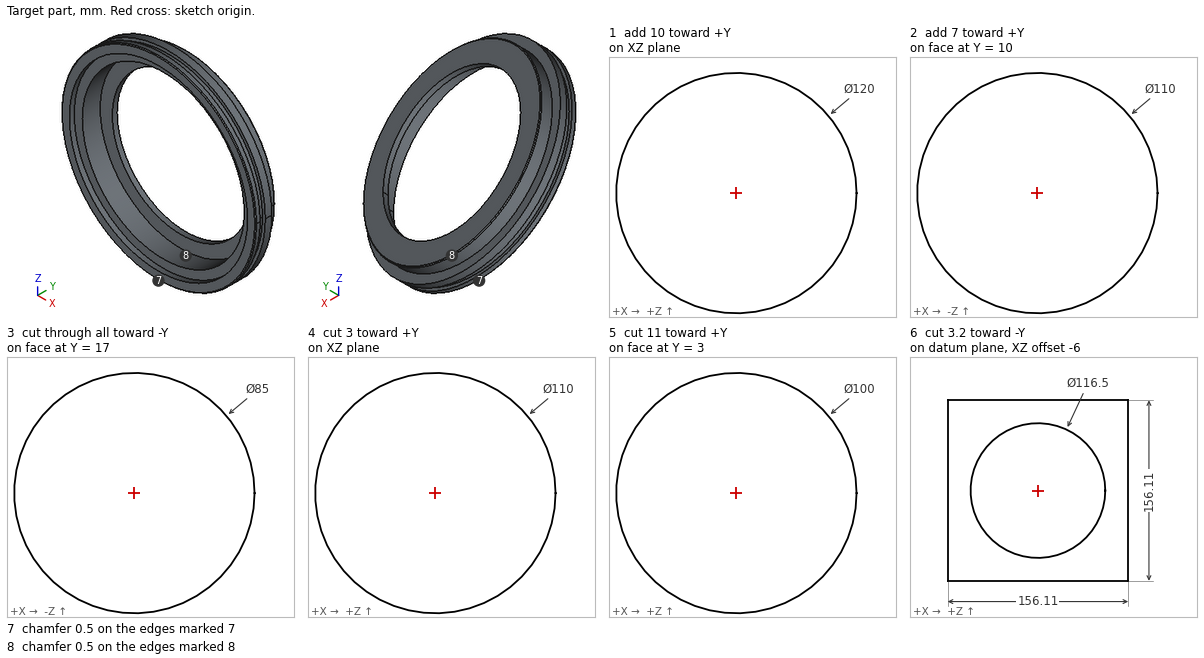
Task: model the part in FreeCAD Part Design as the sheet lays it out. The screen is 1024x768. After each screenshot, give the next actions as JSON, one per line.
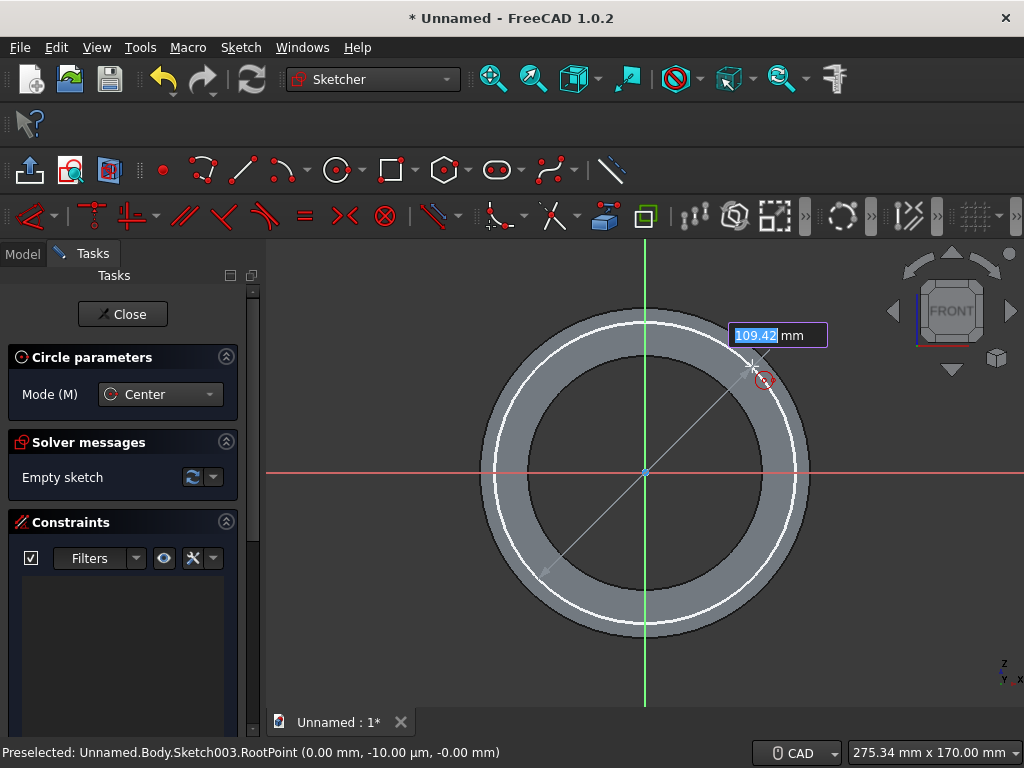
{"action": "type", "text": "110"}
{"action": "key", "text": "Return"}
{"action": "key", "text": "Escape"}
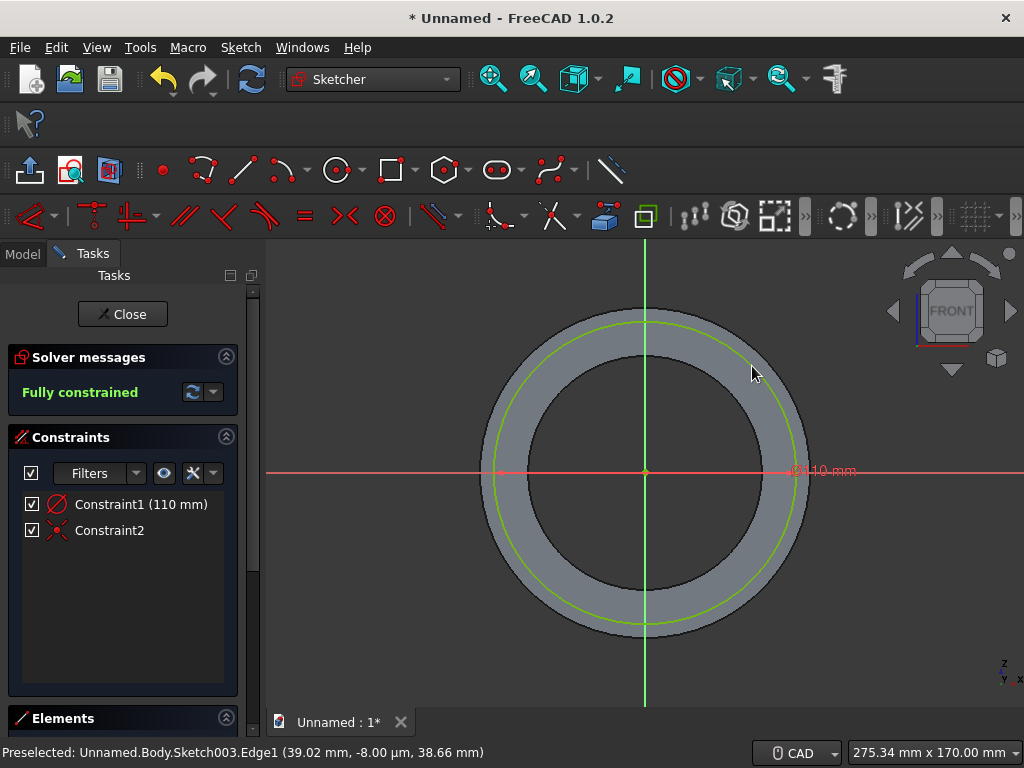
{"action": "left_click", "coordinate": [123, 314]}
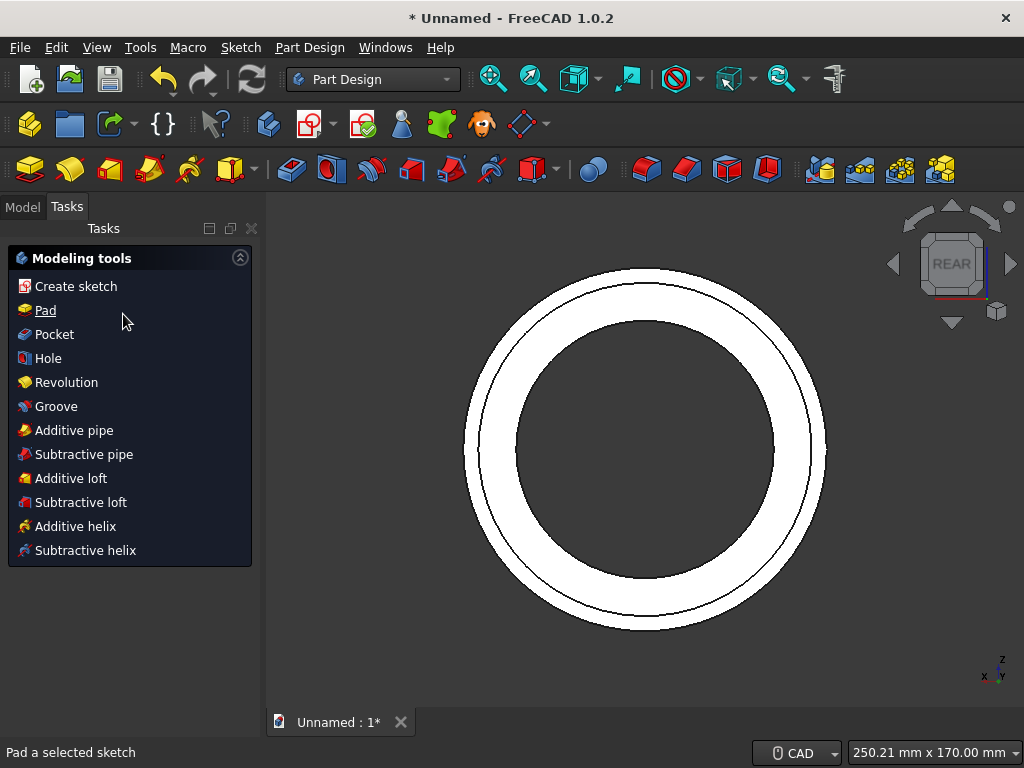
{"action": "left_click", "coordinate": [292, 170]}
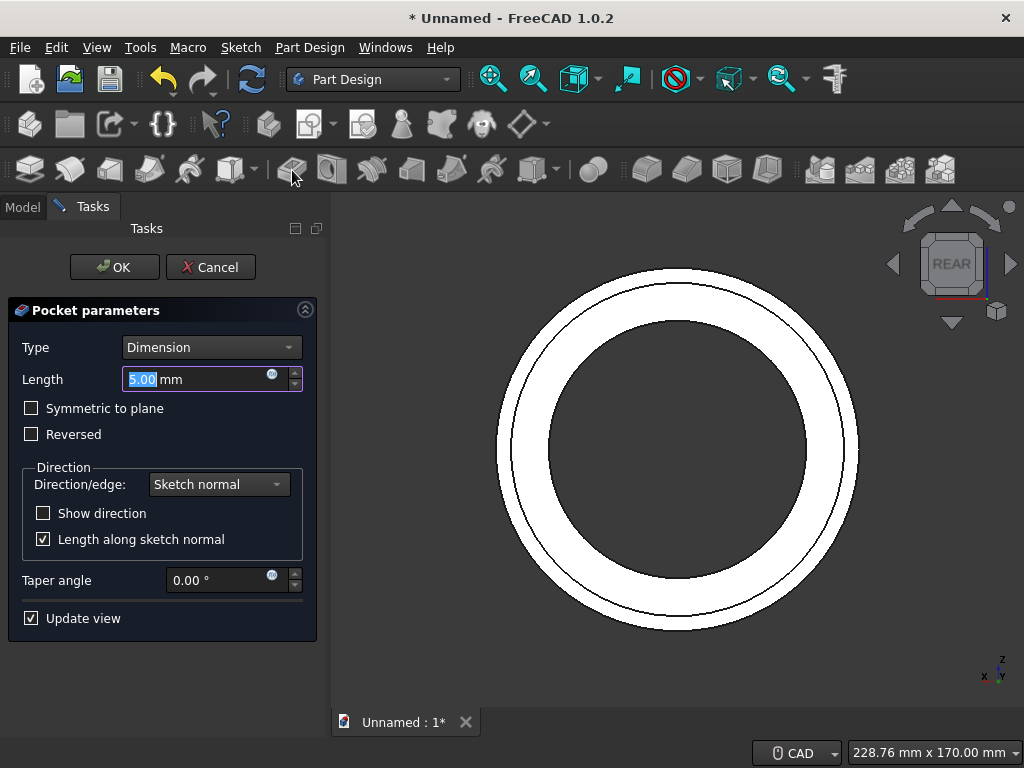
{"action": "type", "text": "3"}
{"action": "key", "text": "Tab"}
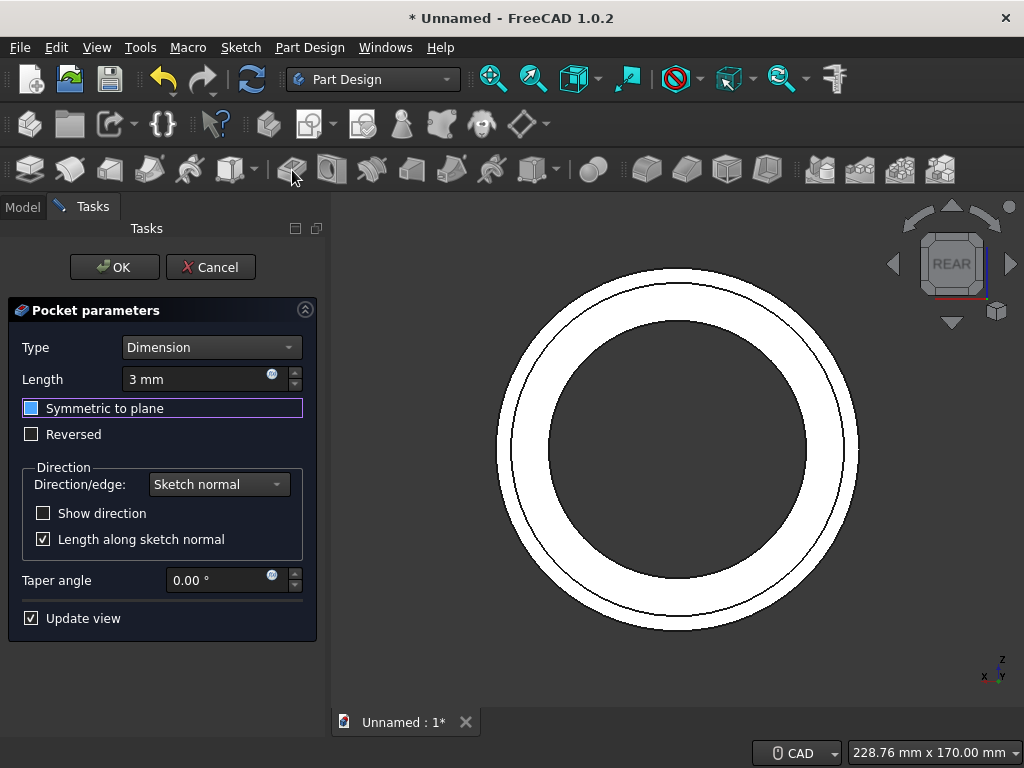
{"action": "left_click", "coordinate": [115, 267]}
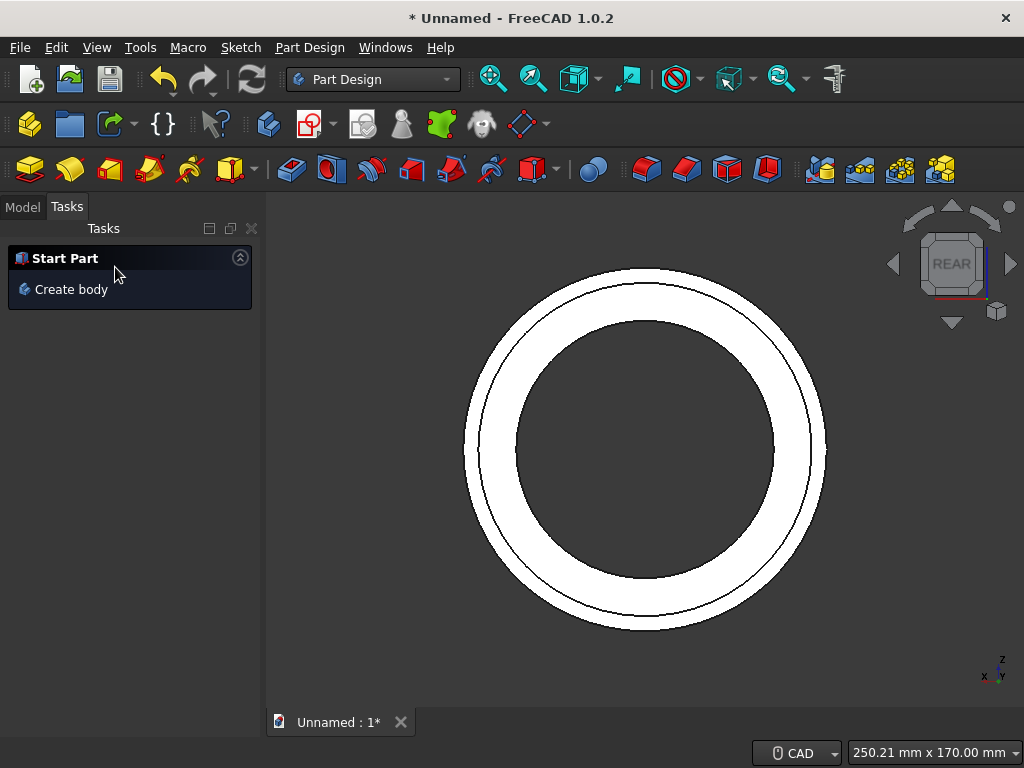
{"action": "key", "text": "0"}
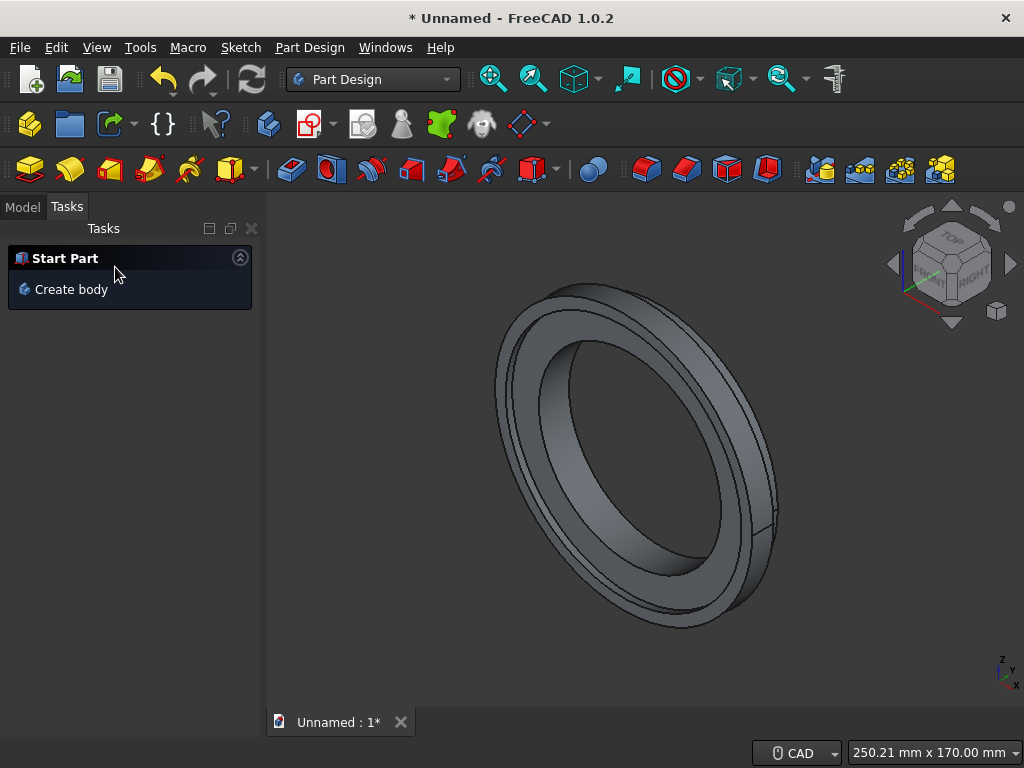
{"action": "left_click", "coordinate": [664, 593]}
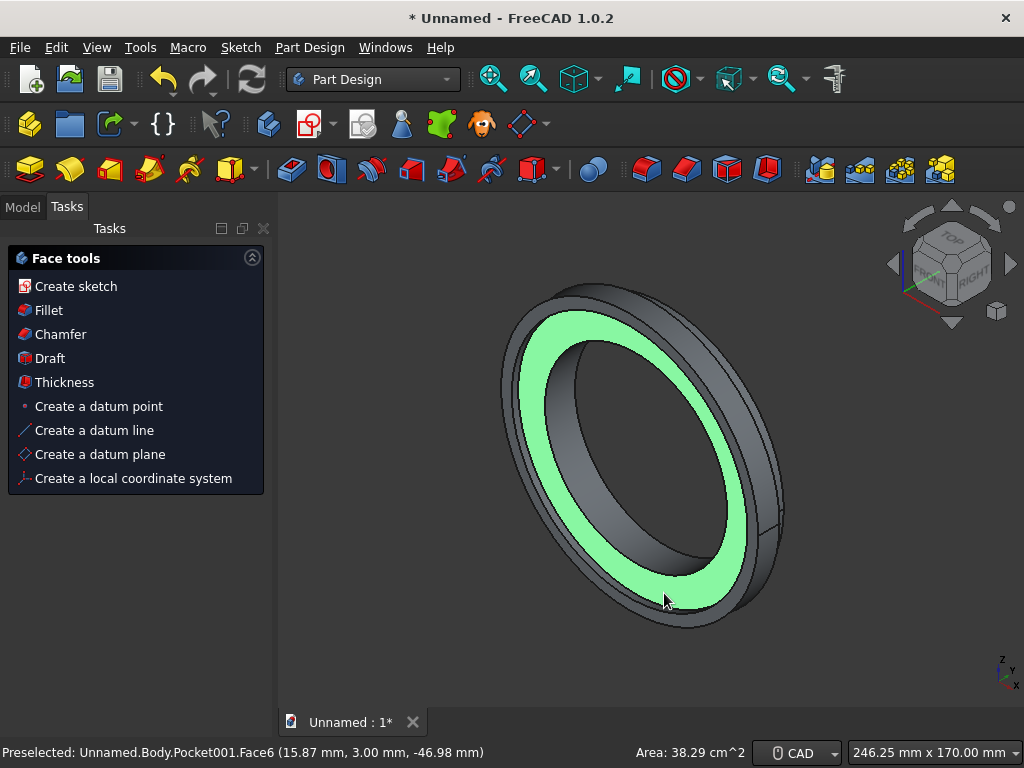
{"action": "left_click", "coordinate": [310, 124]}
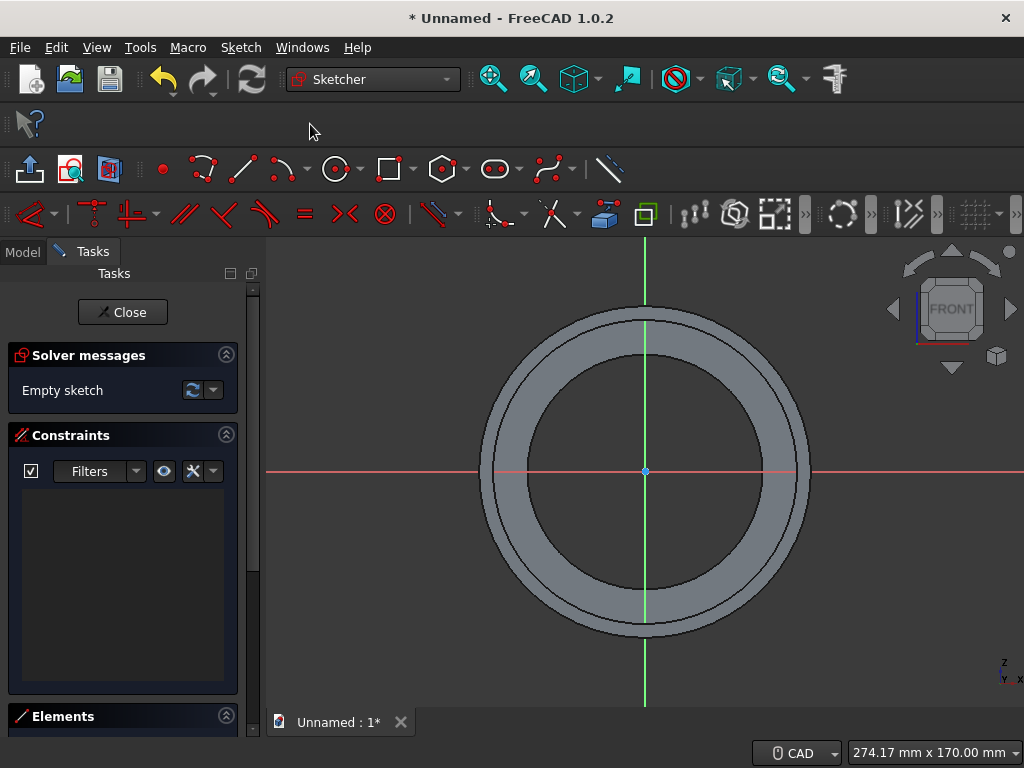
{"action": "key", "text": "g c"}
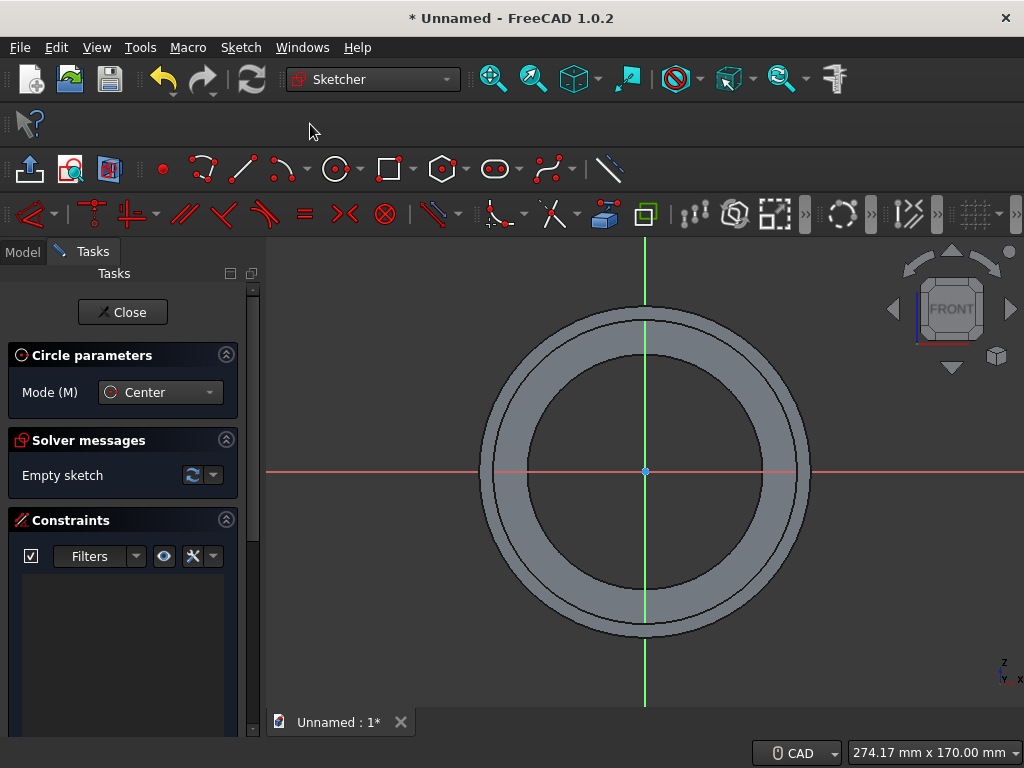
{"action": "left_click", "coordinate": [645, 472]}
{"action": "mouse_move", "coordinate": [743, 374]}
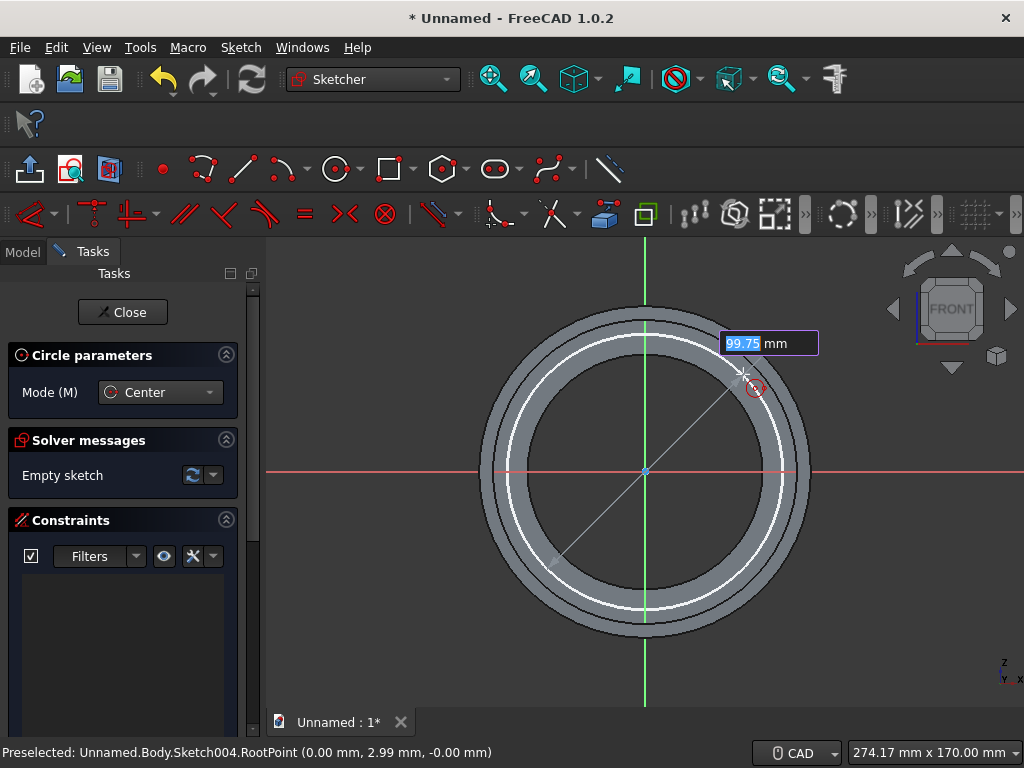
{"action": "type", "text": "100"}
{"action": "key", "text": "Return"}
{"action": "key", "text": "Escape"}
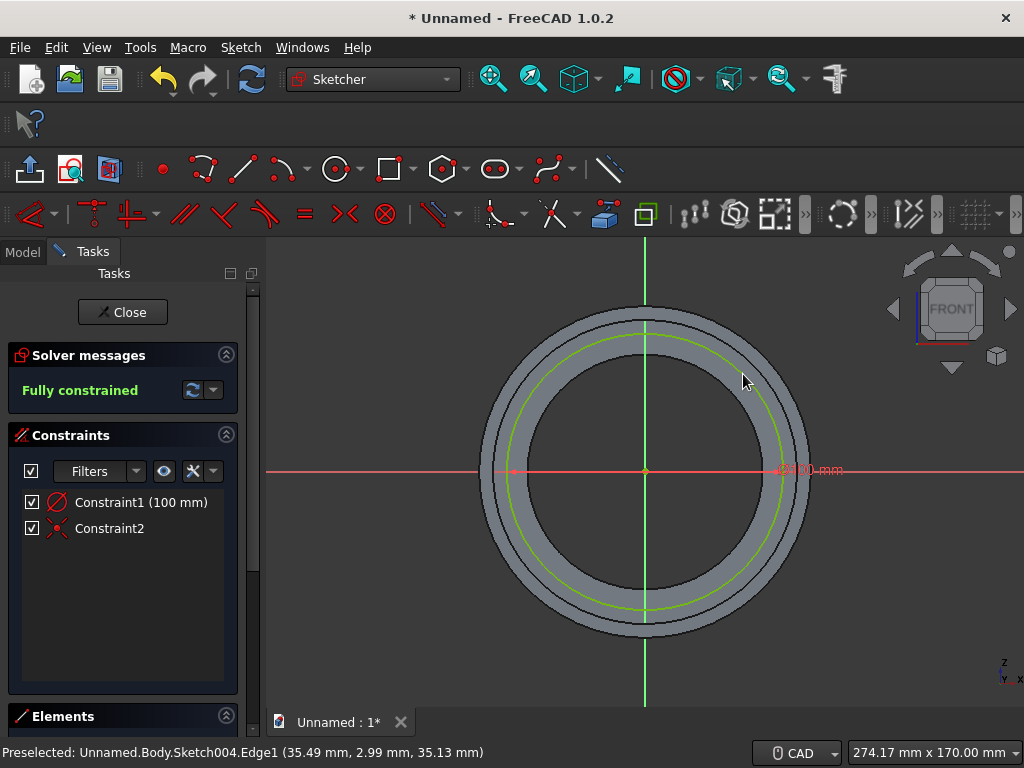
{"action": "left_click", "coordinate": [123, 312]}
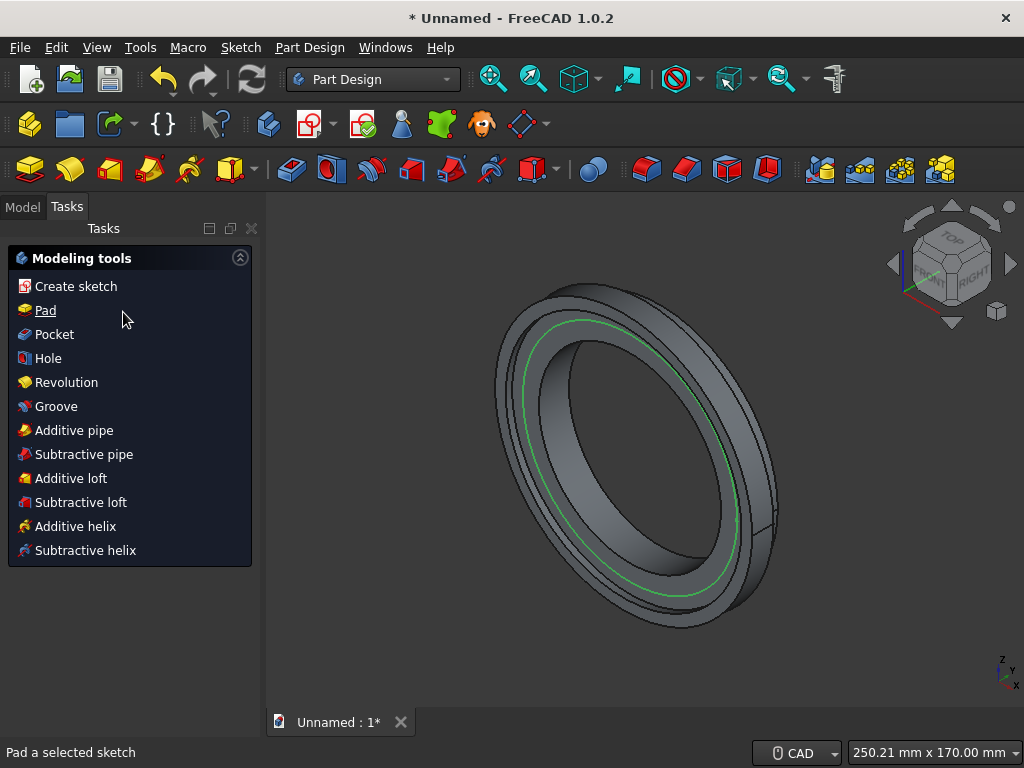
{"action": "left_click", "coordinate": [292, 170]}